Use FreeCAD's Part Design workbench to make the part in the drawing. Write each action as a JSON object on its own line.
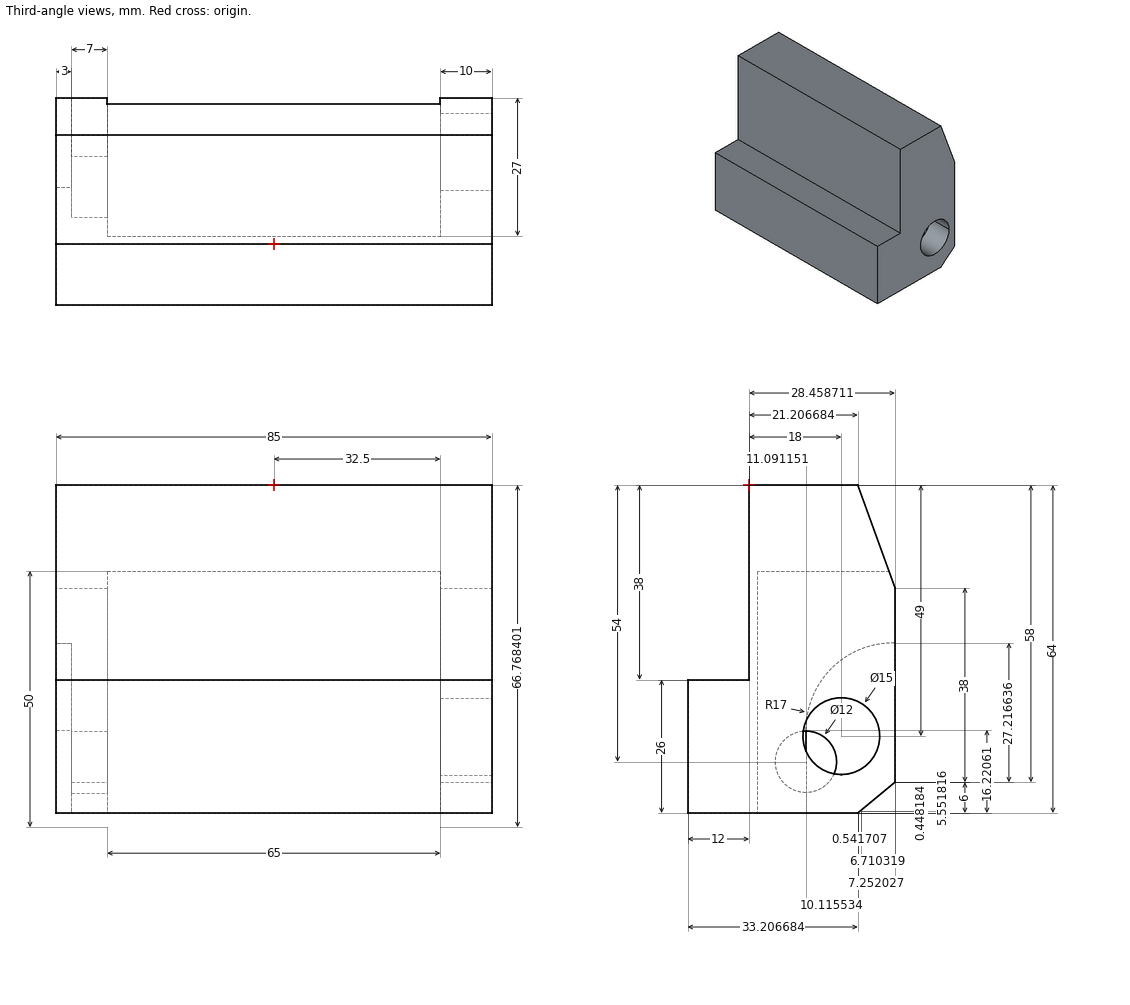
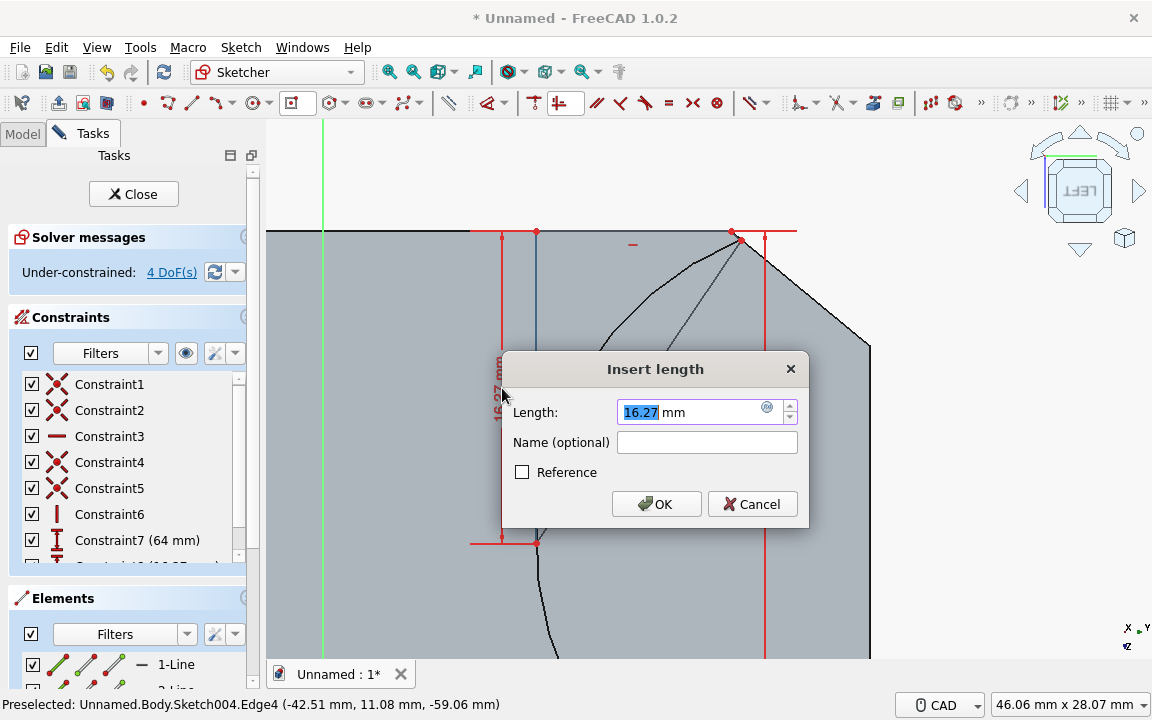
{"action": "type", "text": "16.22061"}
{"action": "key", "text": "Return"}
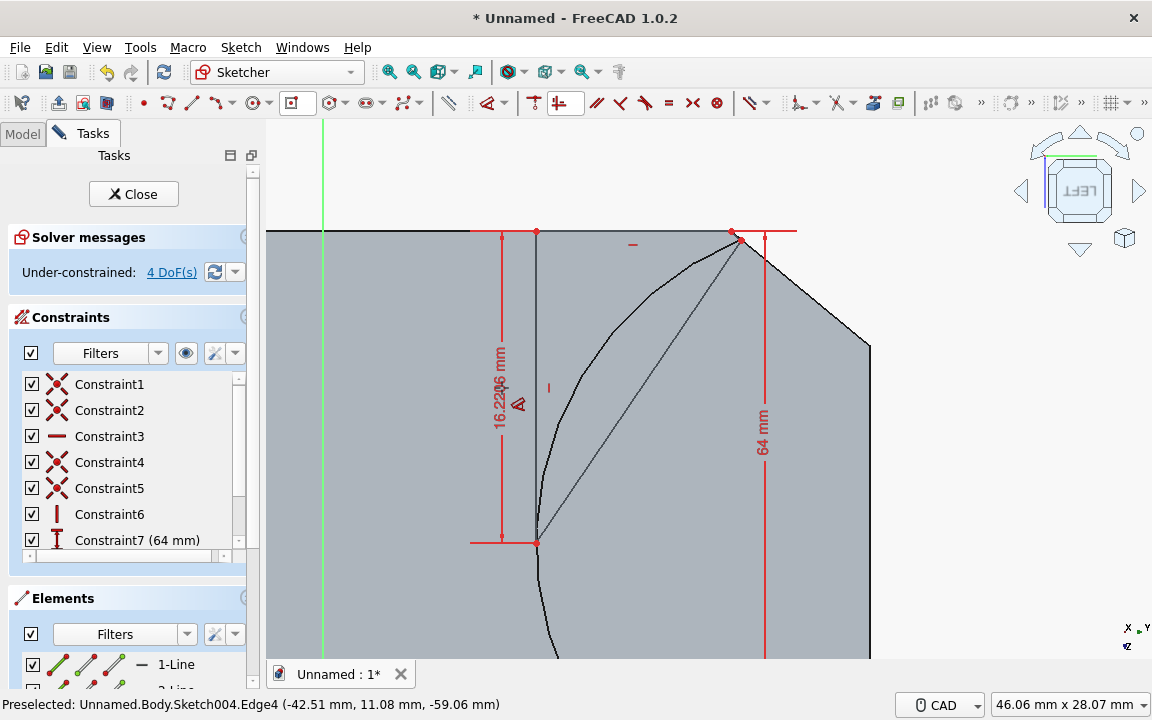
{"action": "left_click", "coordinate": [672, 231]}
{"action": "left_click", "coordinate": [633, 197]}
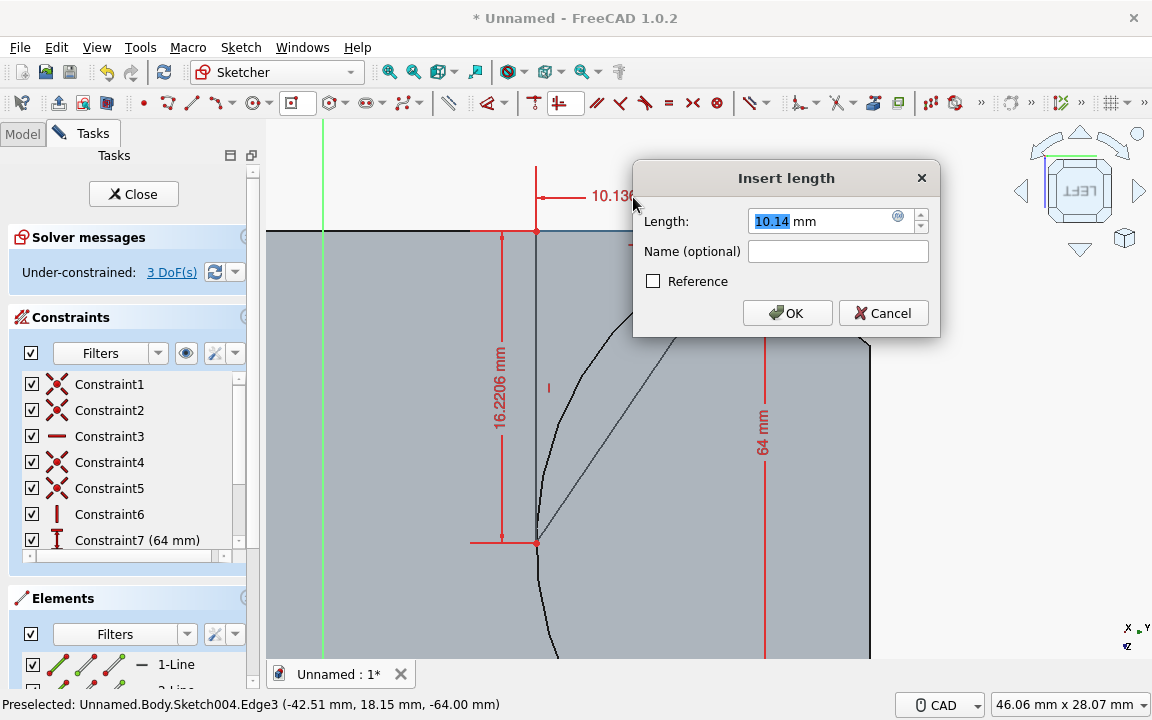
{"action": "type", "text": "10.115534"}
{"action": "key", "text": "Return"}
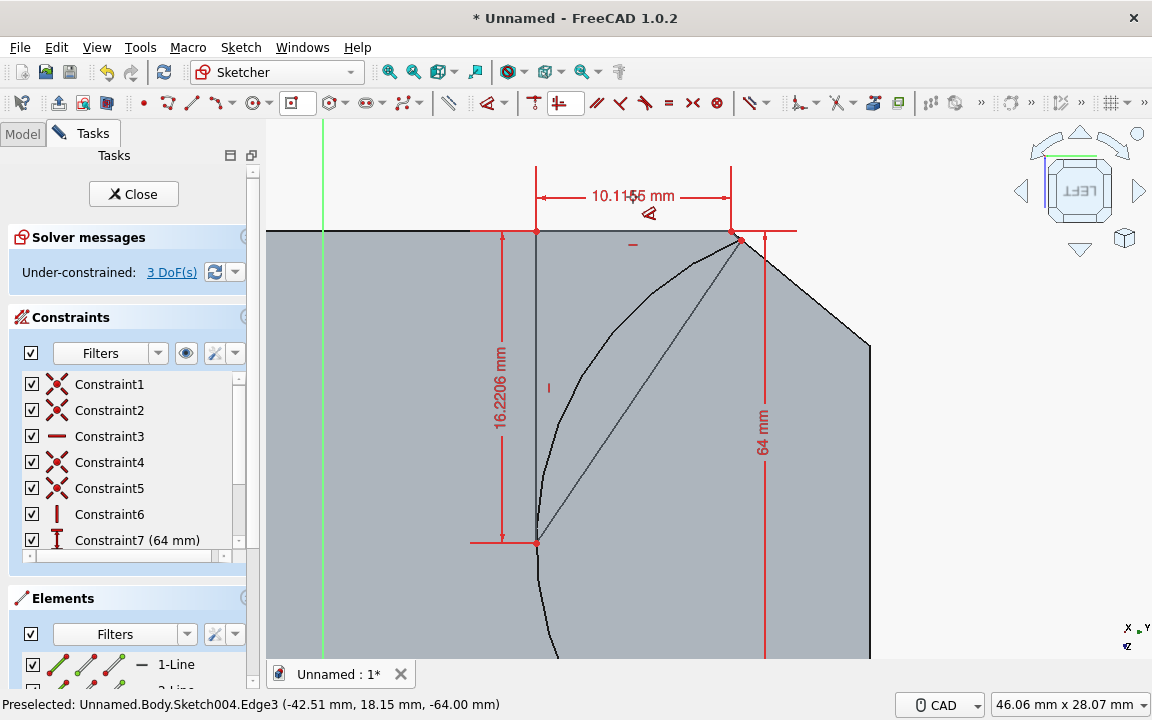
{"action": "scroll", "coordinate": [736, 236], "scroll_direction": "up", "scroll_amount": 7}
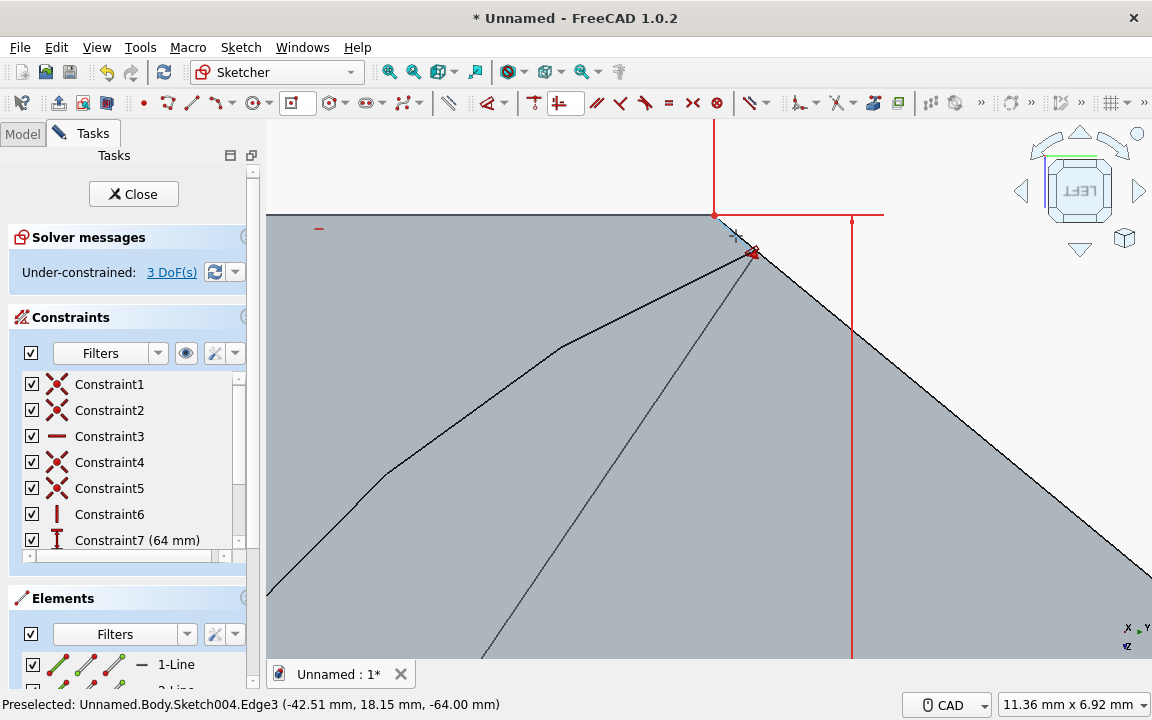
{"action": "left_click", "coordinate": [734, 235]}
{"action": "left_click", "coordinate": [734, 181]}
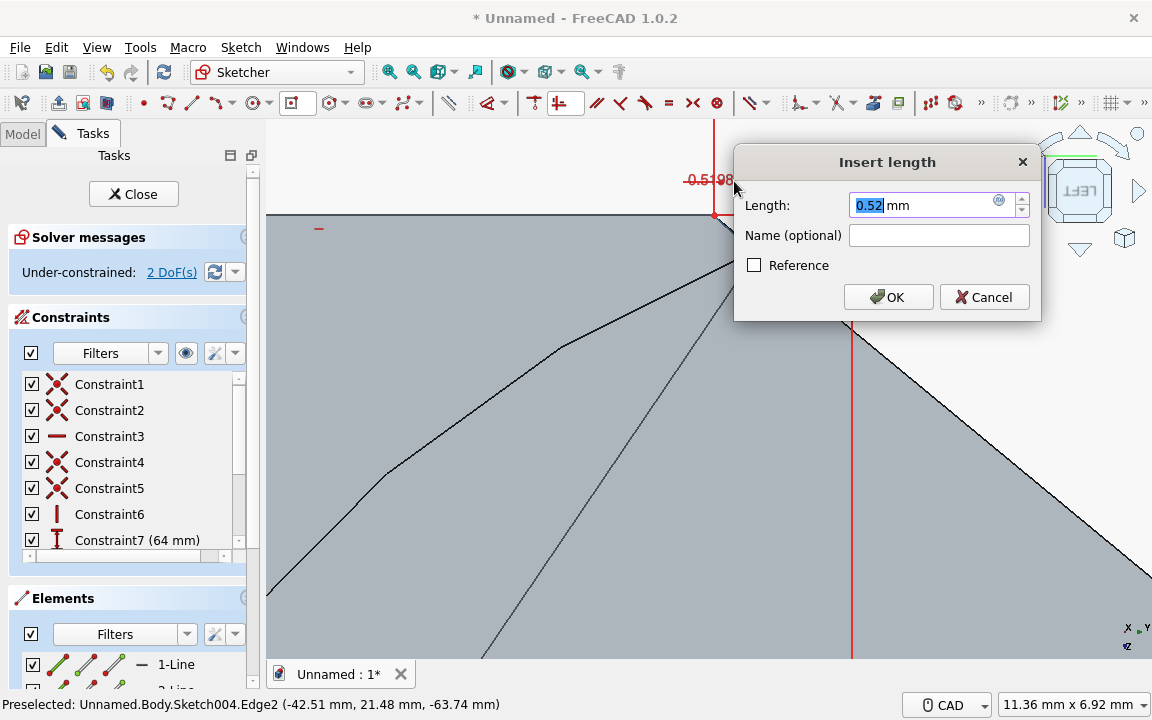
{"action": "type", "text": "0.541707"}
{"action": "key", "text": "Return"}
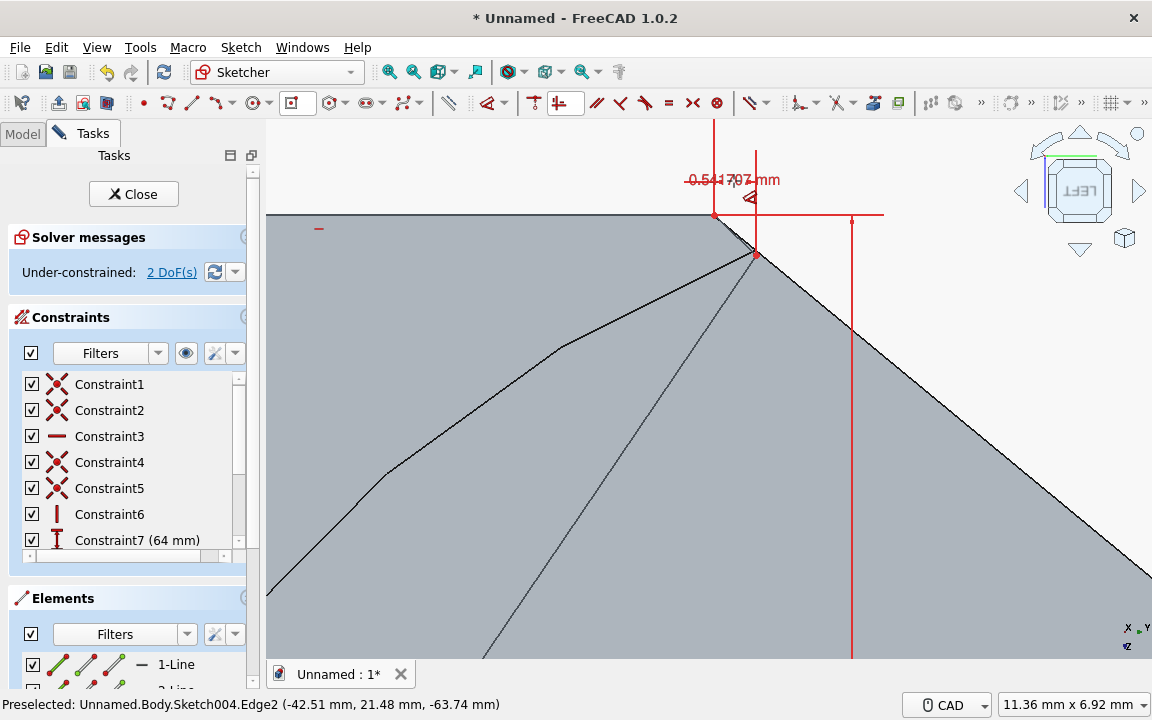
{"action": "left_click", "coordinate": [744, 243]}
{"action": "left_click", "coordinate": [790, 235]}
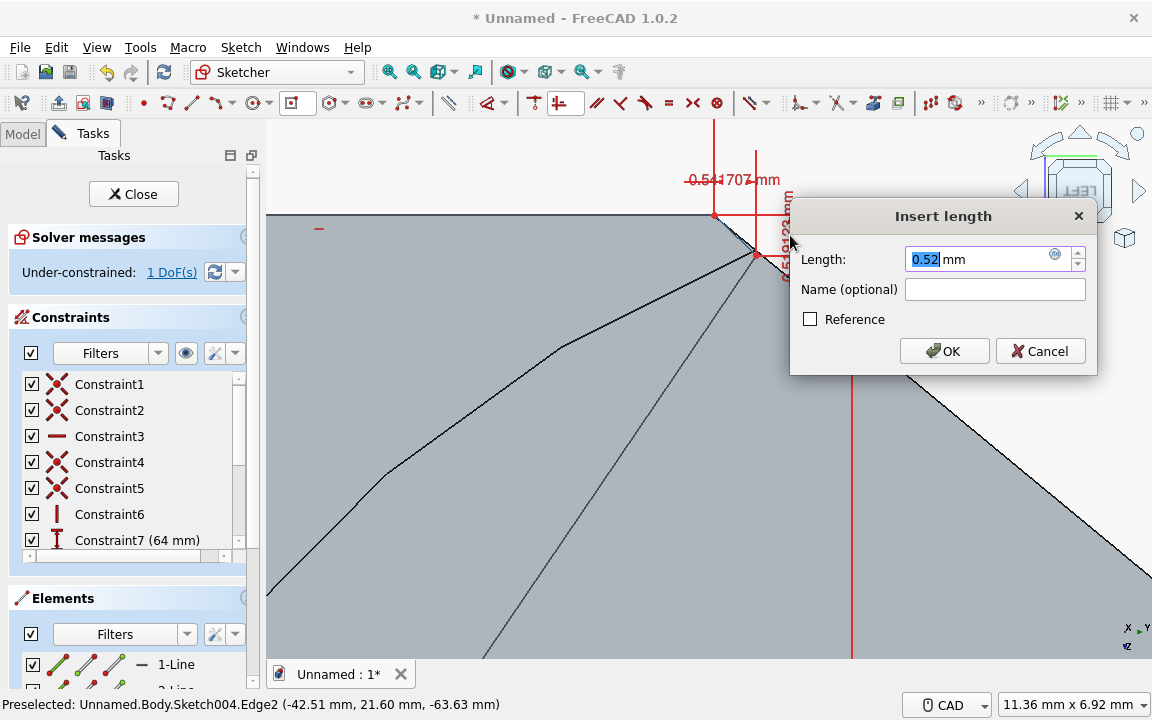
{"action": "type", "text": "0.448184"}
{"action": "key", "text": "Return"}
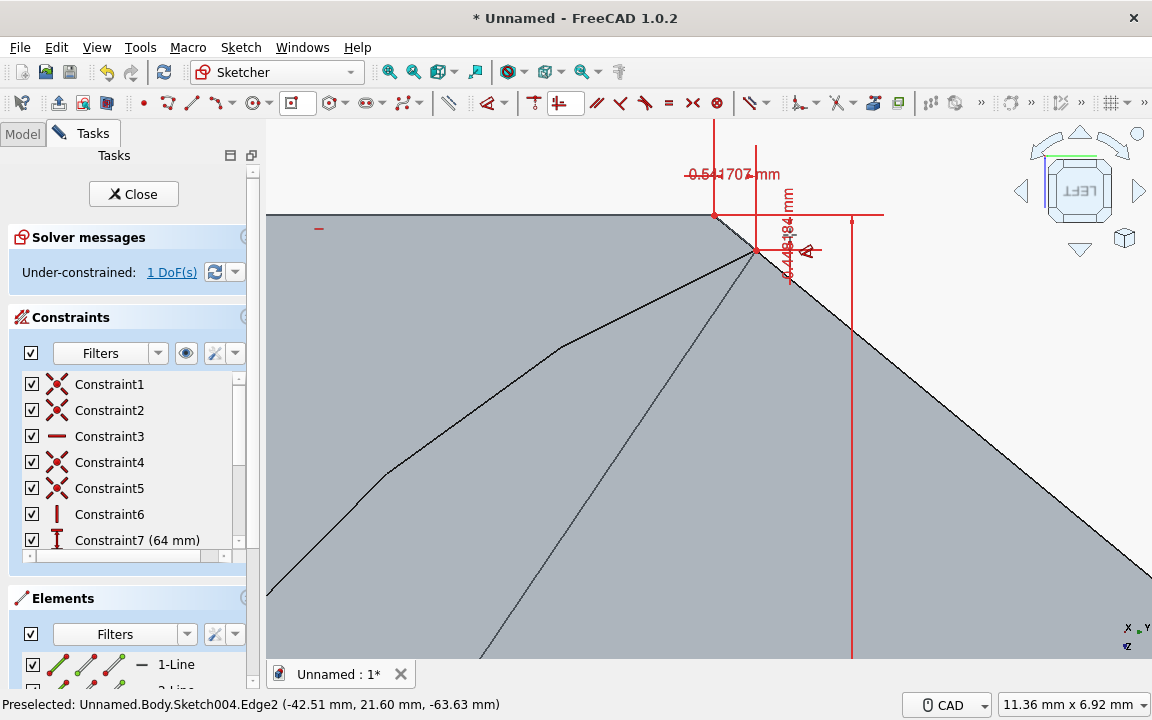
{"action": "scroll", "coordinate": [739, 239], "scroll_direction": "down", "scroll_amount": 7}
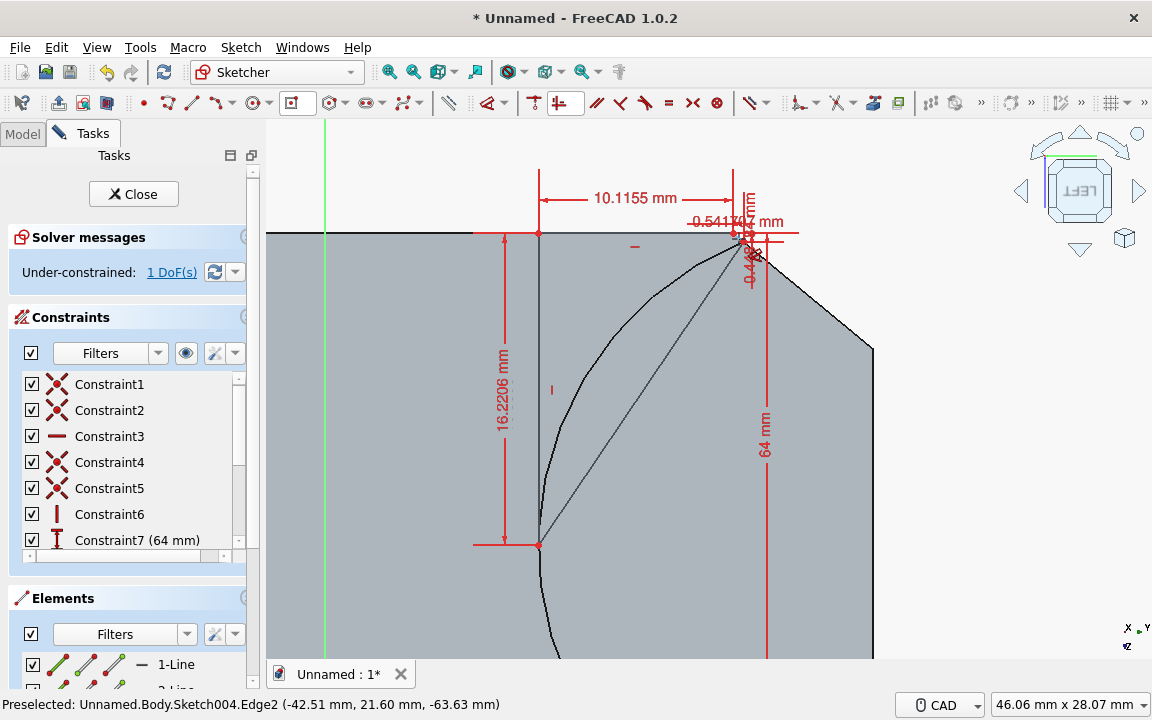
{"action": "left_click", "coordinate": [539, 545]}
{"action": "left_click", "coordinate": [432, 511]}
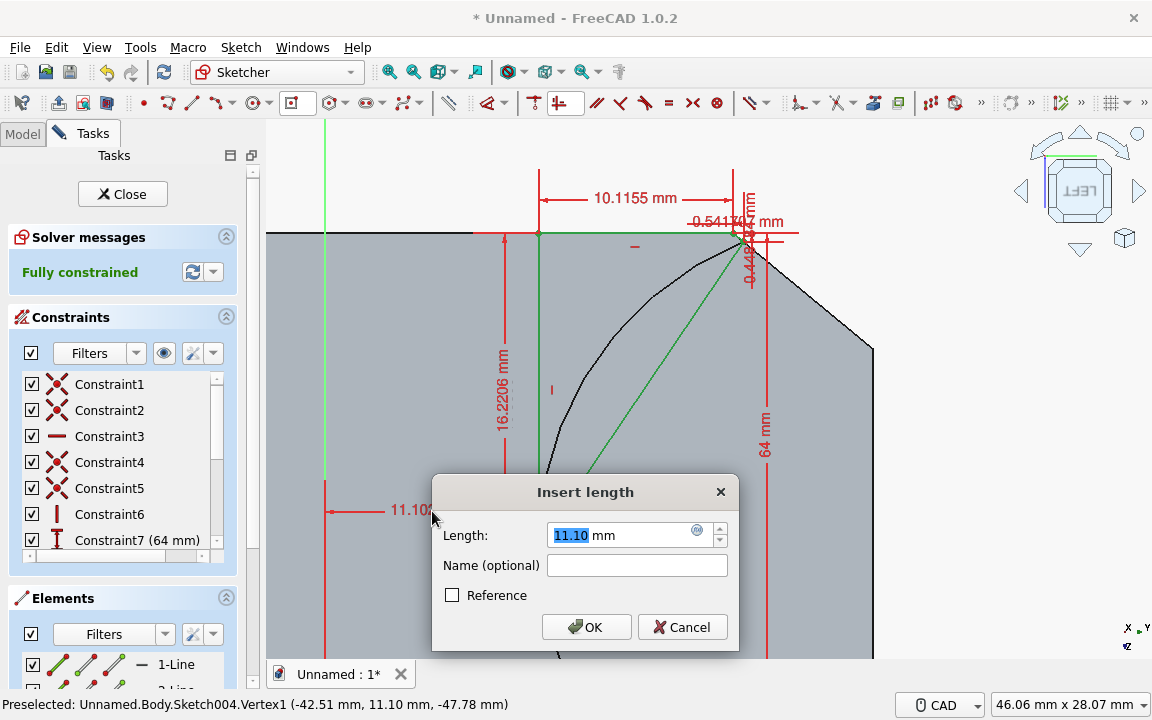
{"action": "type", "text": "11.091151"}
{"action": "key", "text": "Return"}
{"action": "key", "text": "Escape"}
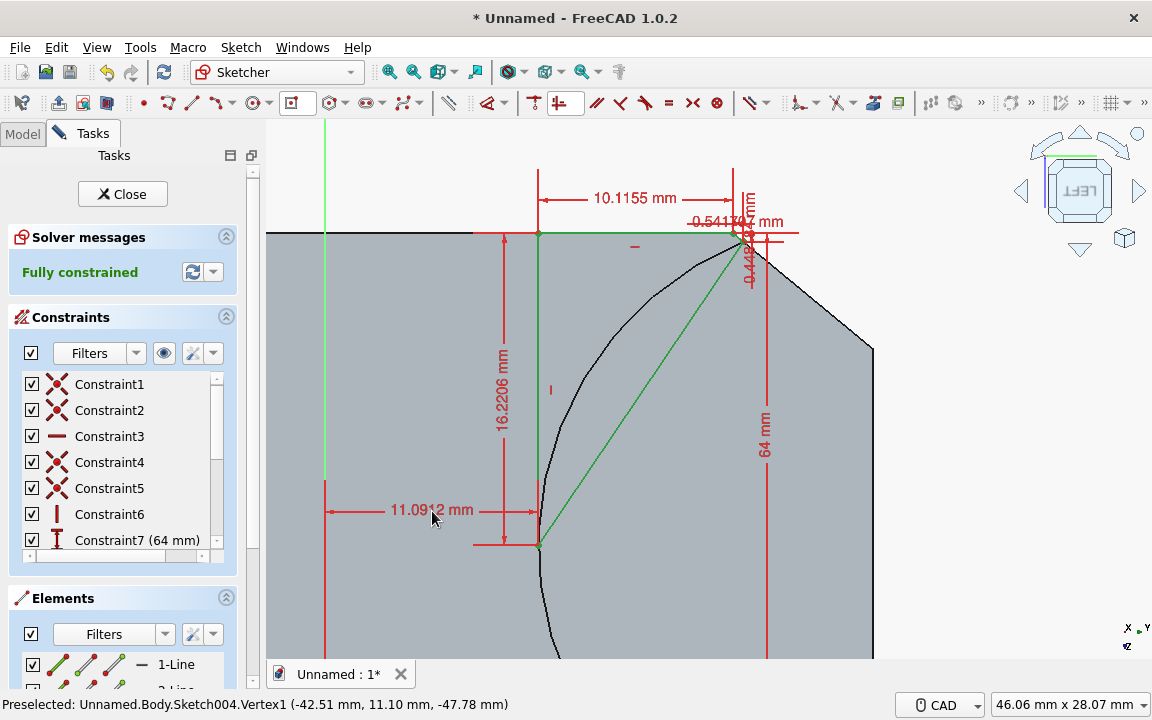
{"action": "left_click", "coordinate": [123, 194]}